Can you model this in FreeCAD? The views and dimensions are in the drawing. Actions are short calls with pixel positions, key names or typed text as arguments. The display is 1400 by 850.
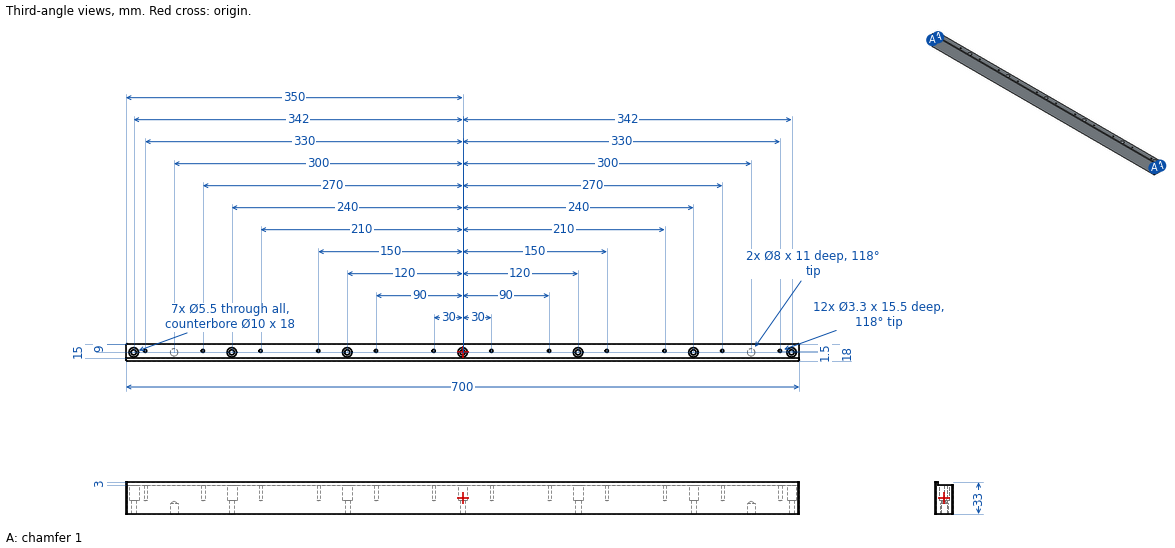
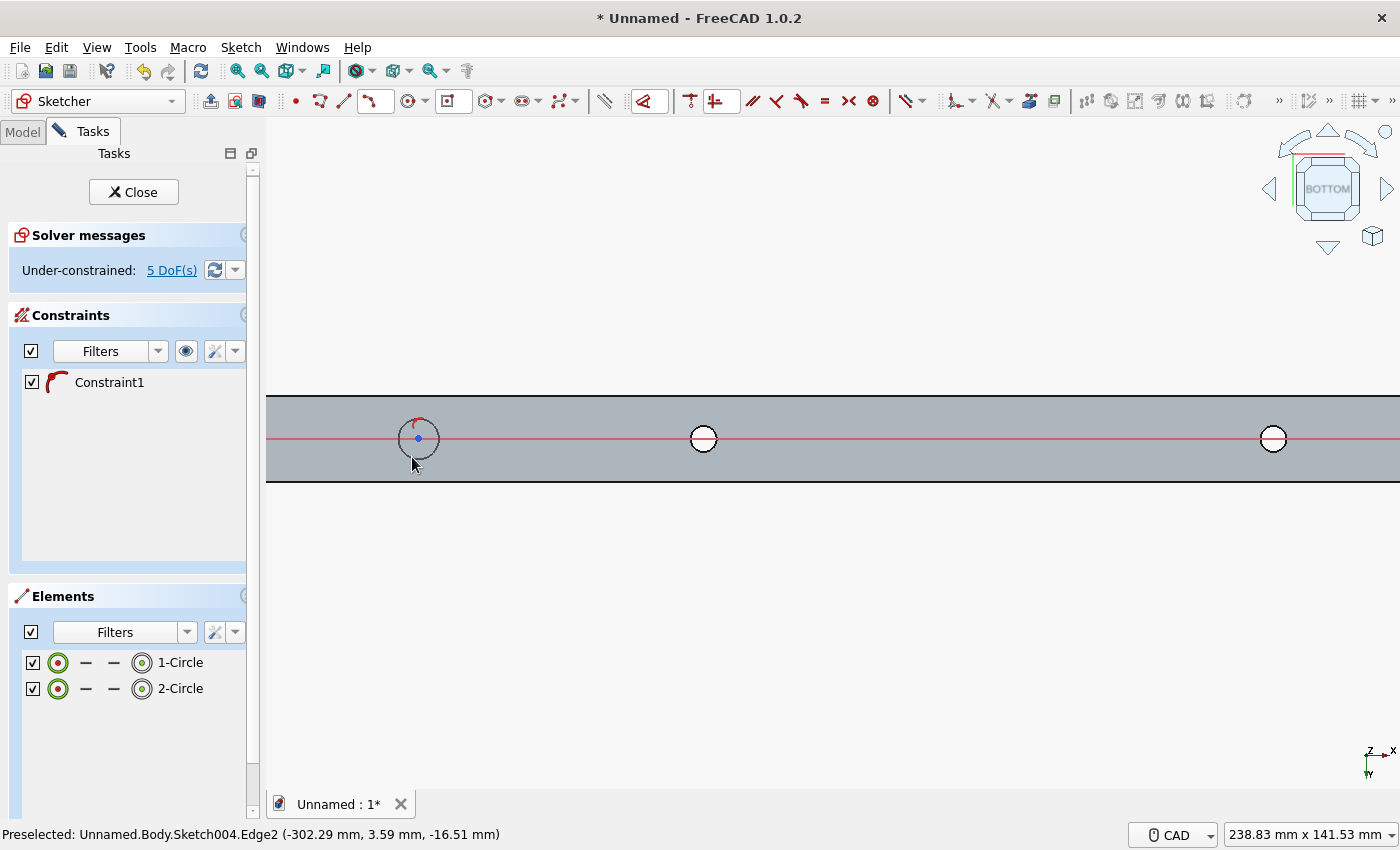
scroll(411, 458, down, 7)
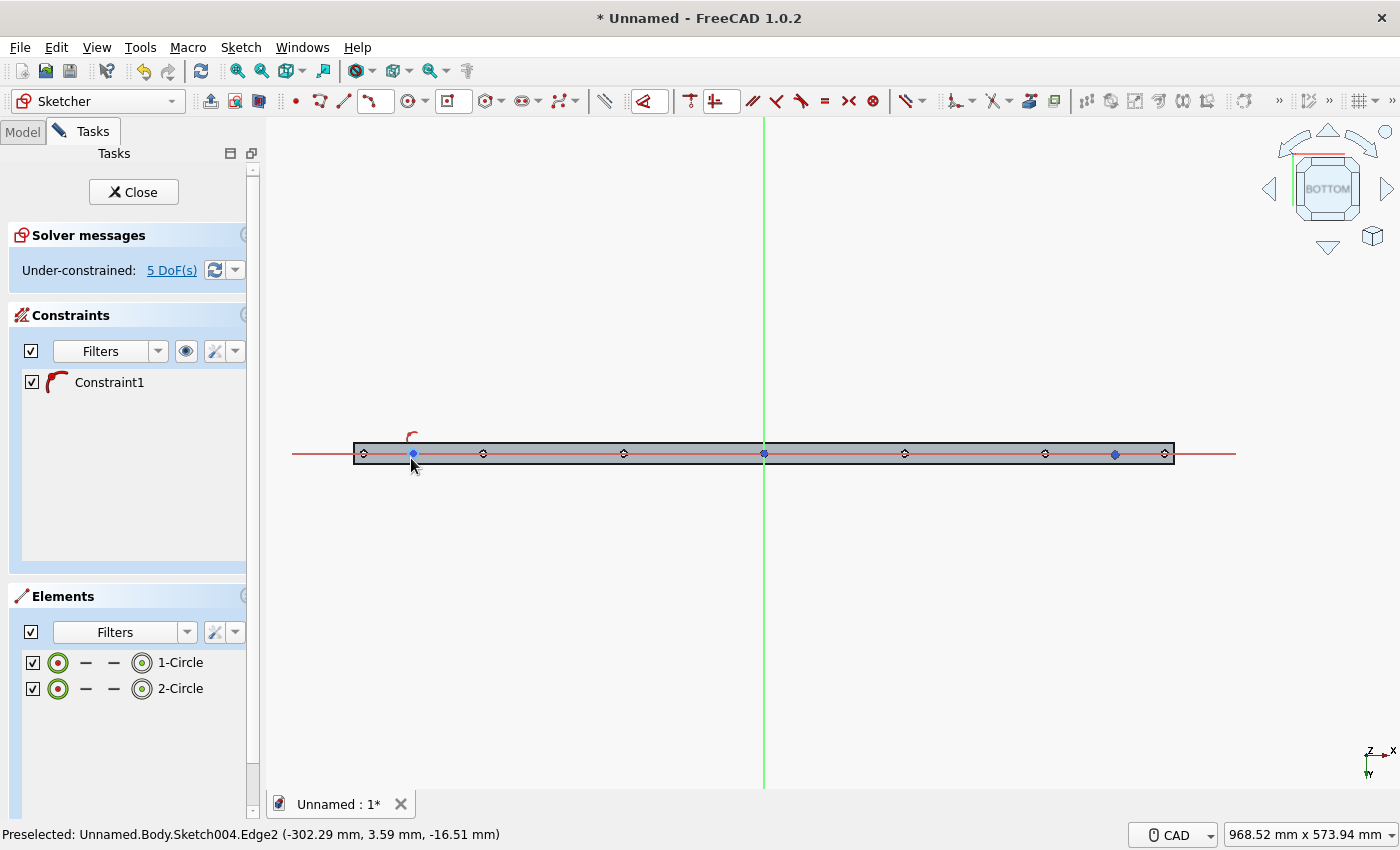
scroll(1113, 458, up, 7)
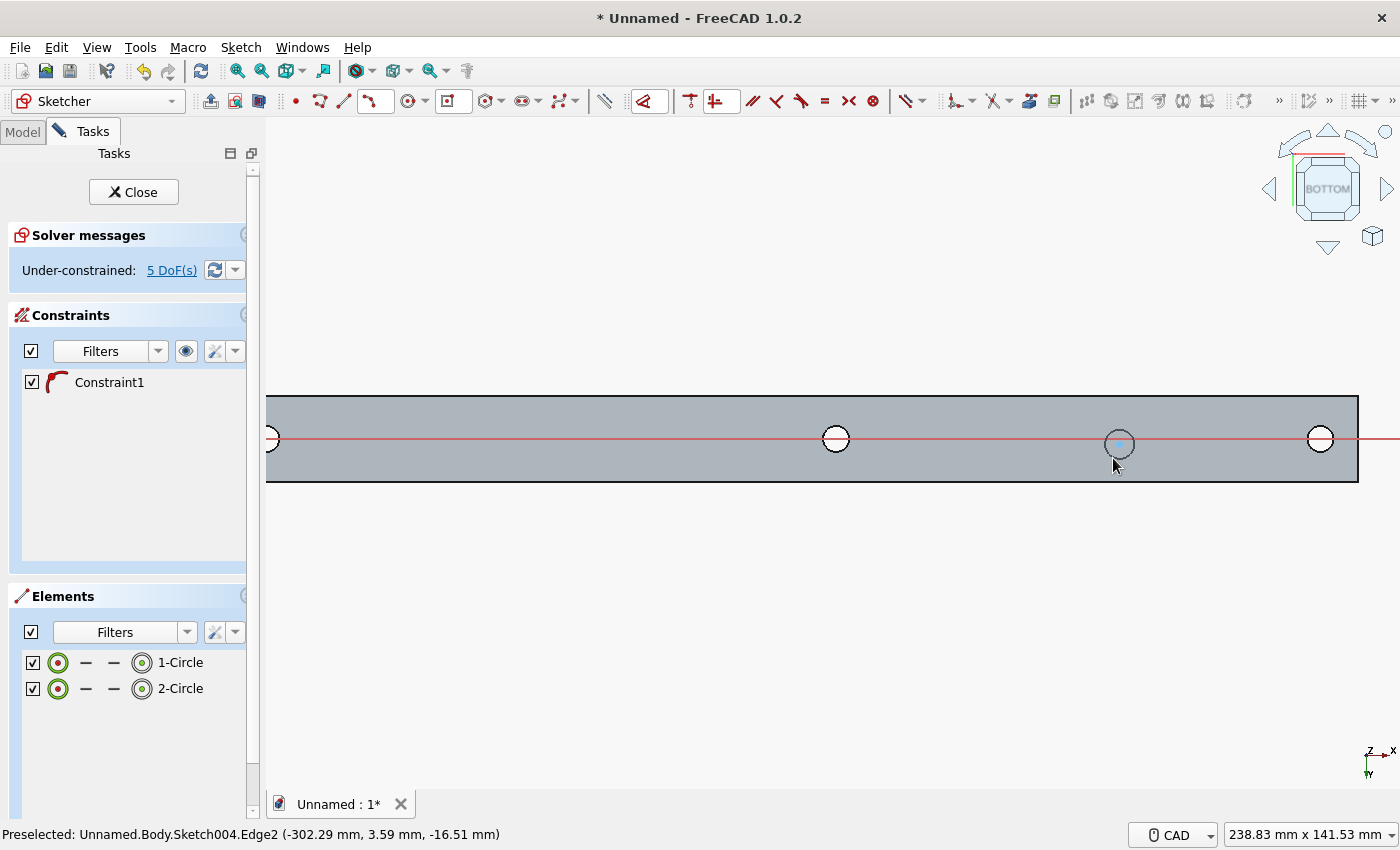
click(1109, 455)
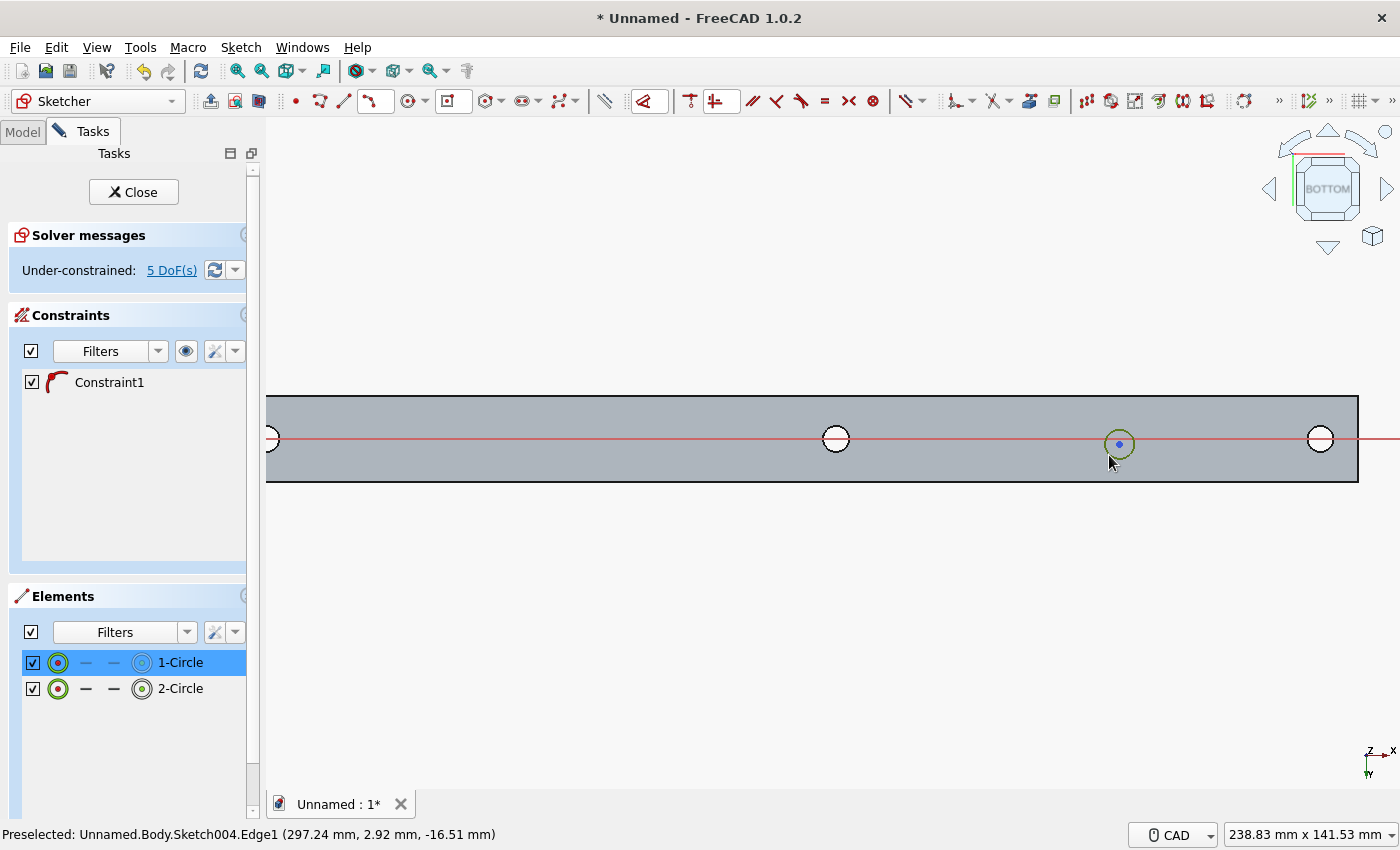
scroll(1114, 458, down, 7)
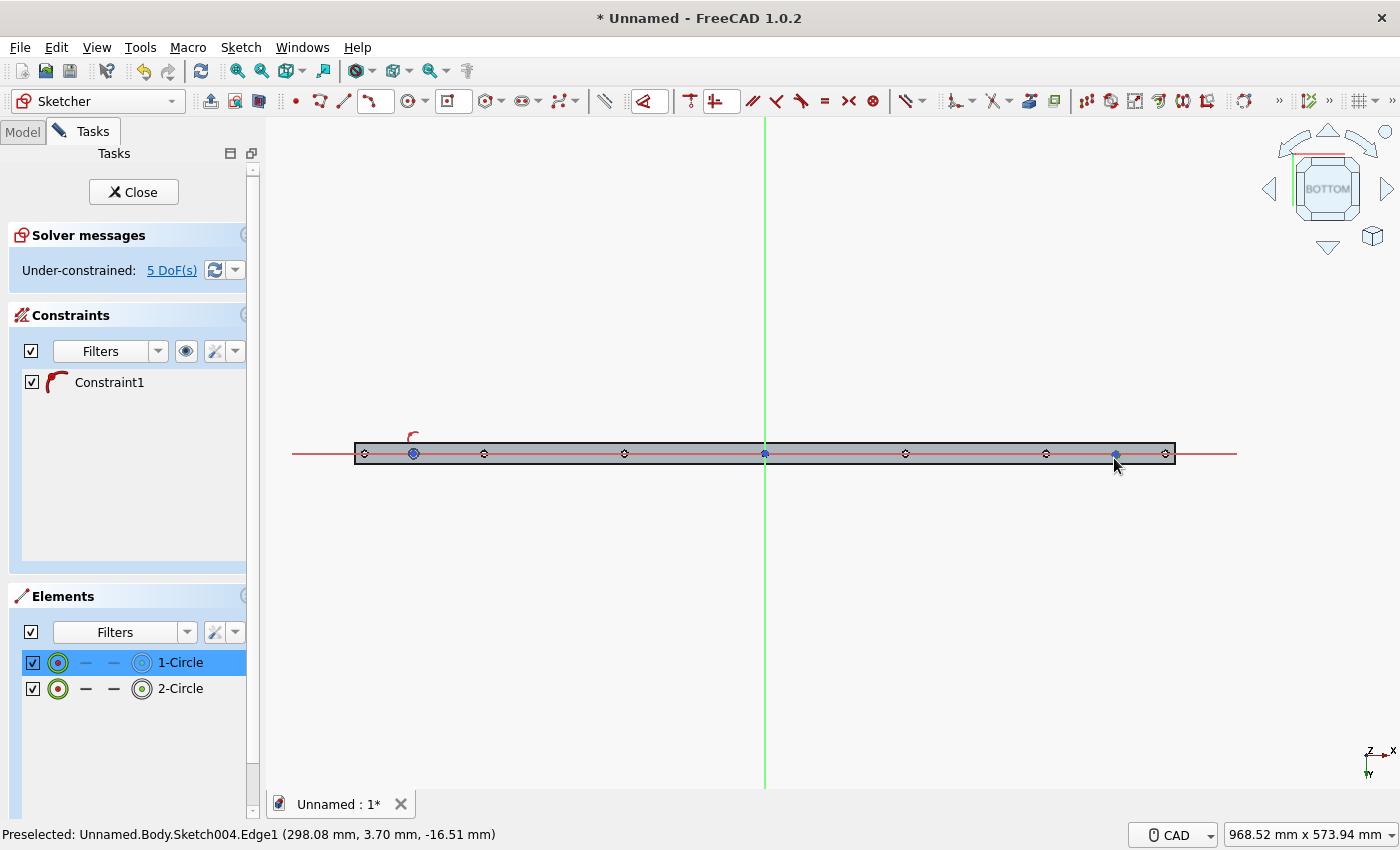
scroll(417, 450, up, 7)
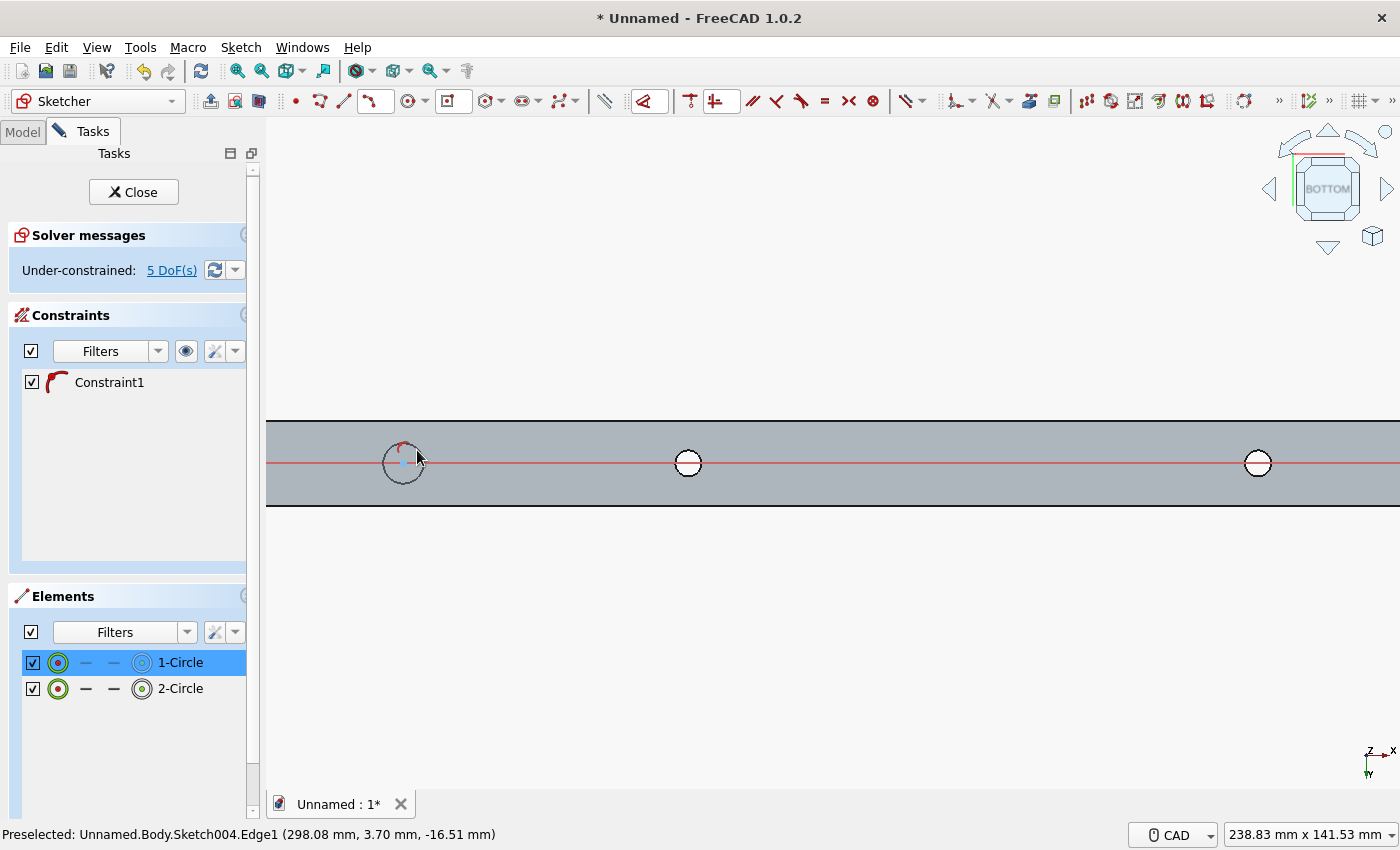
click(418, 449)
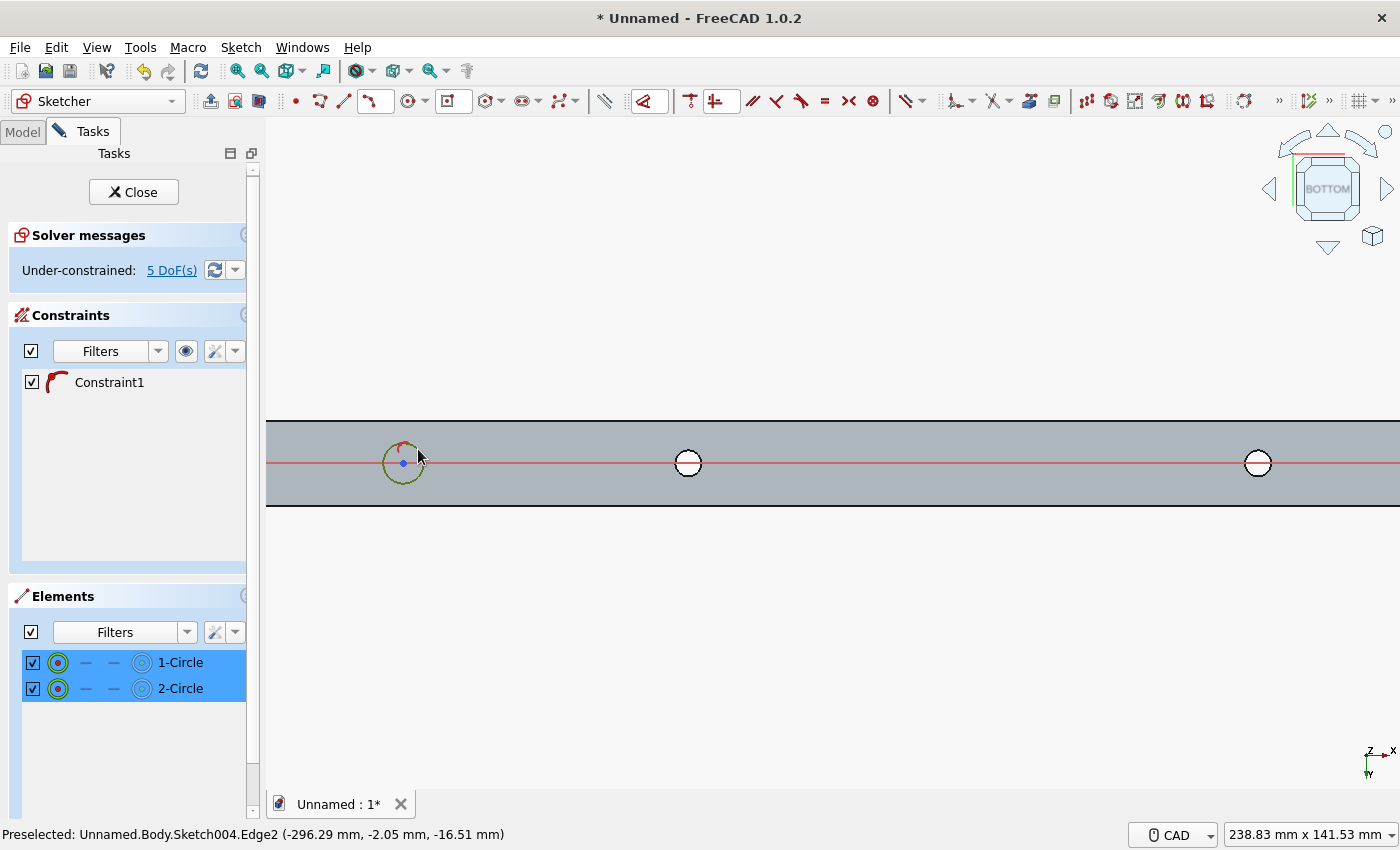
key(e)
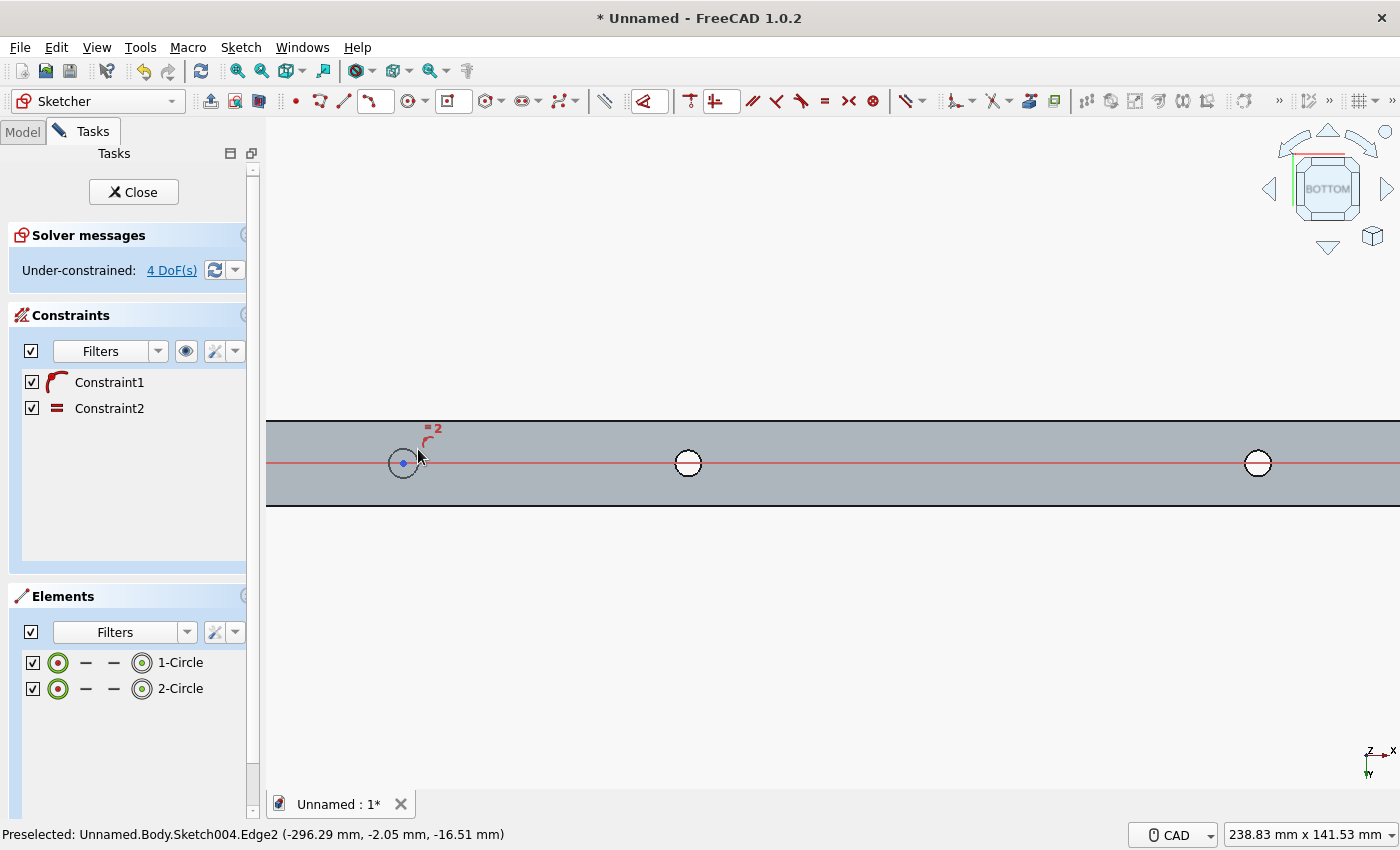
scroll(416, 450, down, 7)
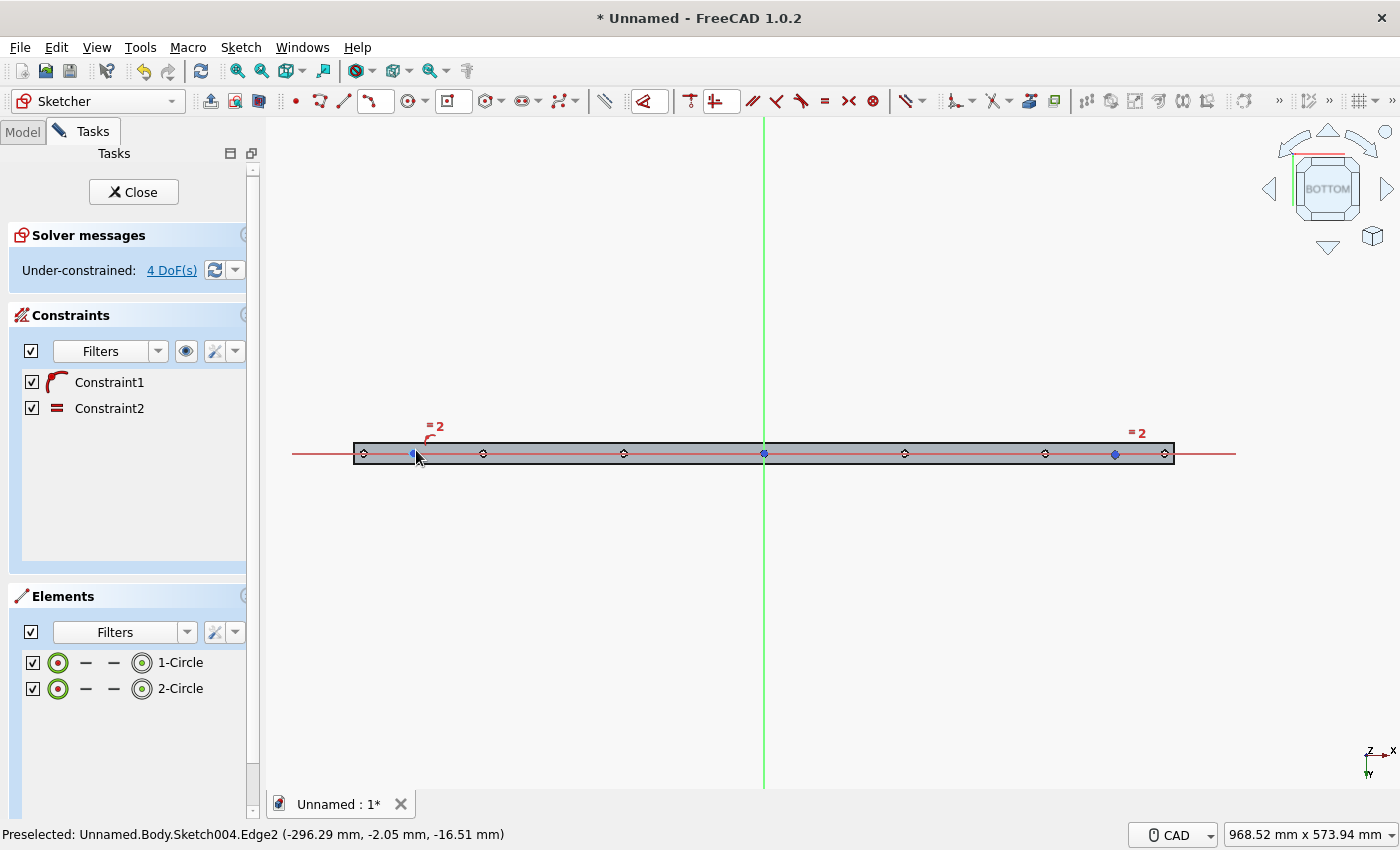
click(1115, 455)